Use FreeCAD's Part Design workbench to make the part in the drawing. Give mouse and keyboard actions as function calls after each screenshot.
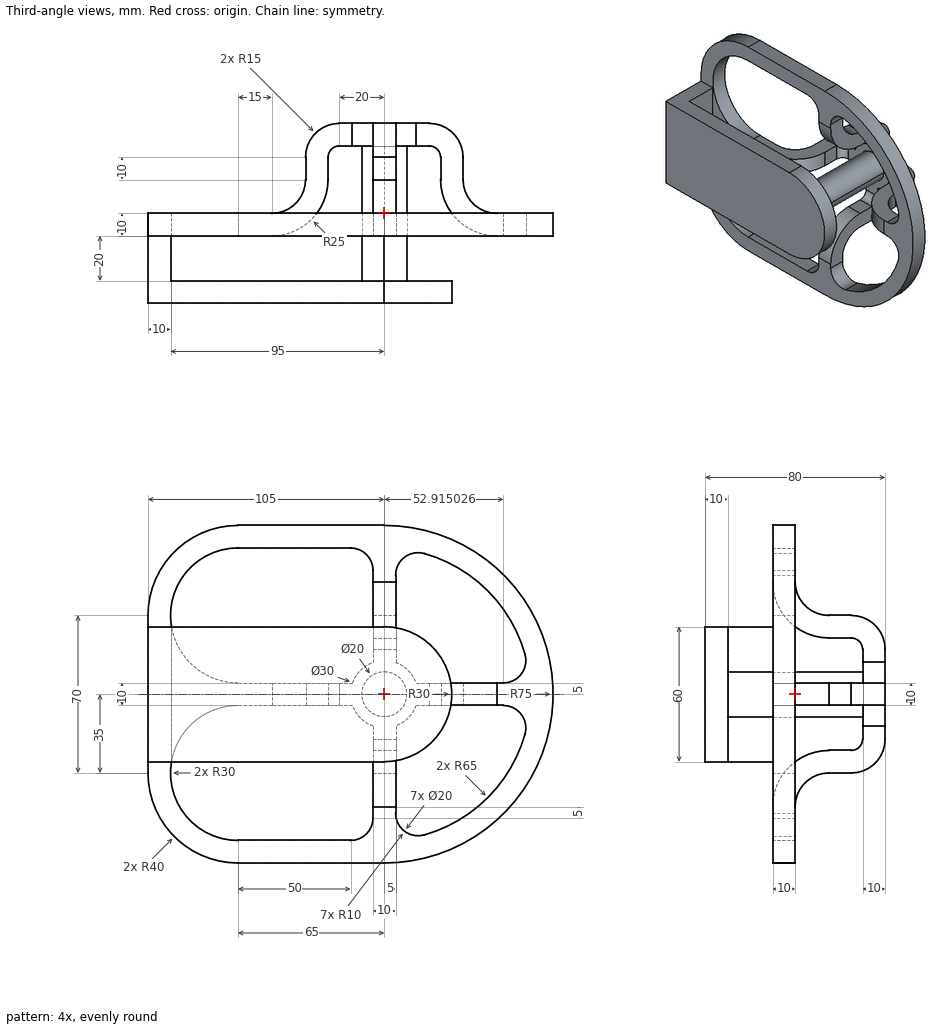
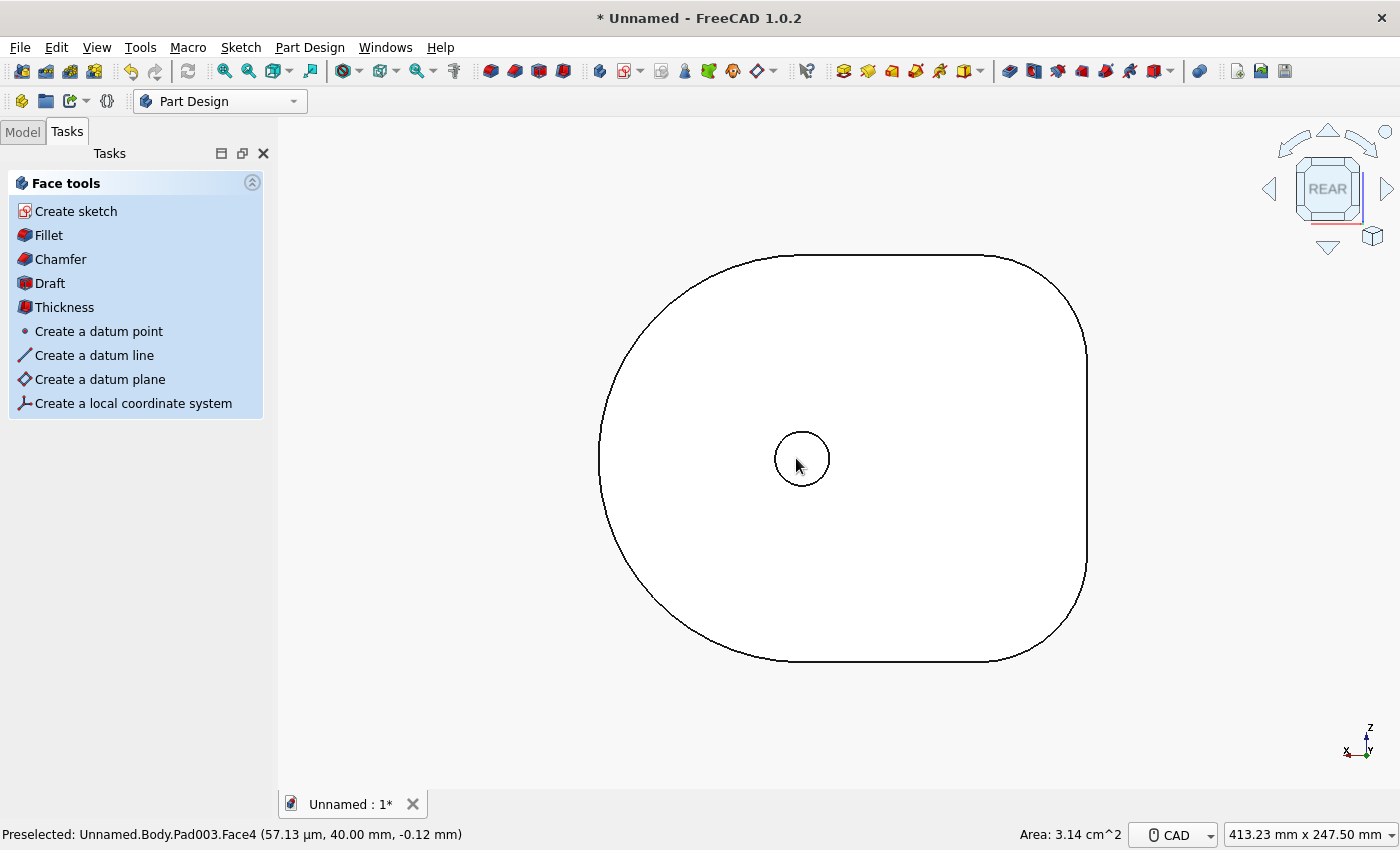
click(624, 72)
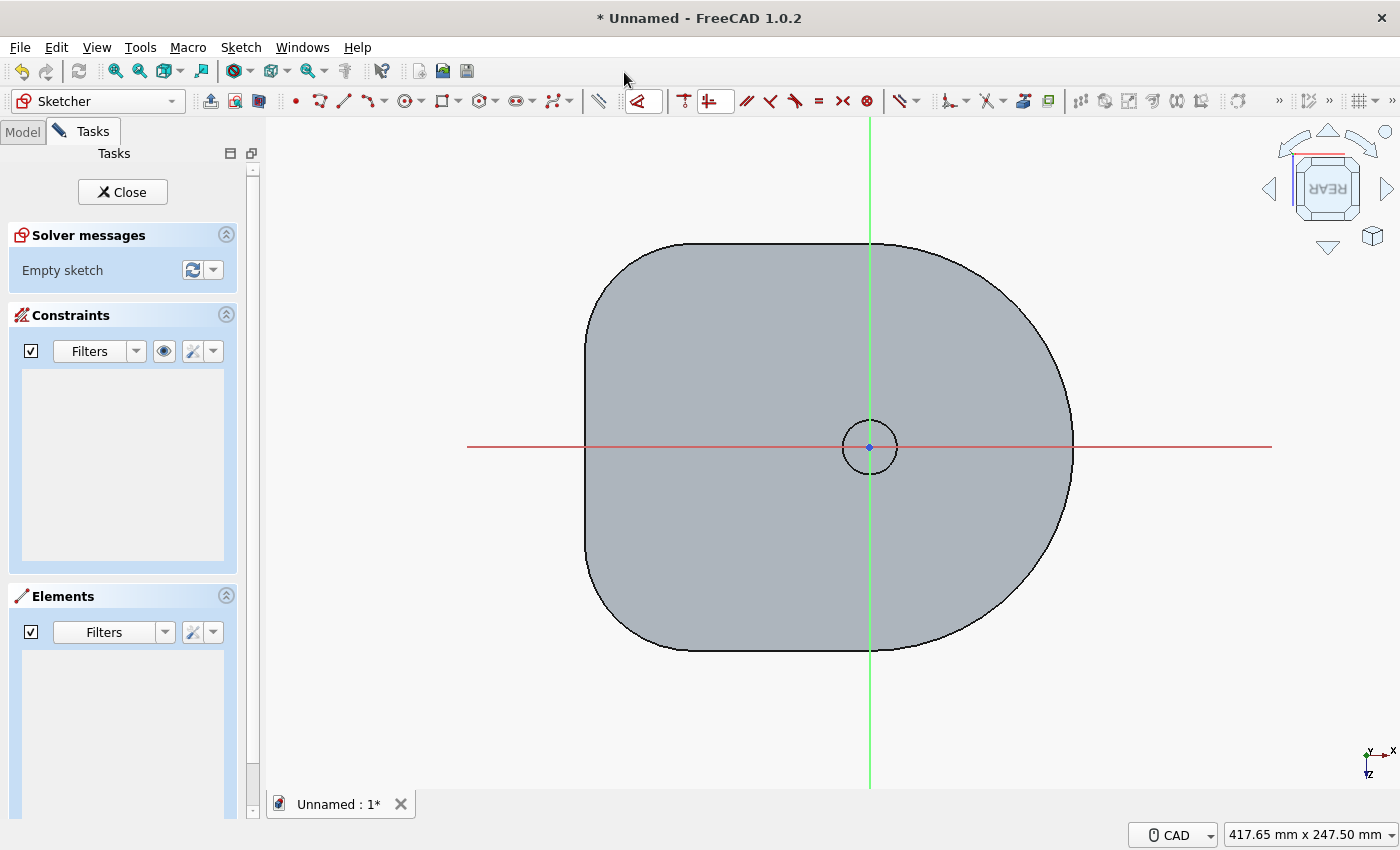
scroll(896, 446, up, 8)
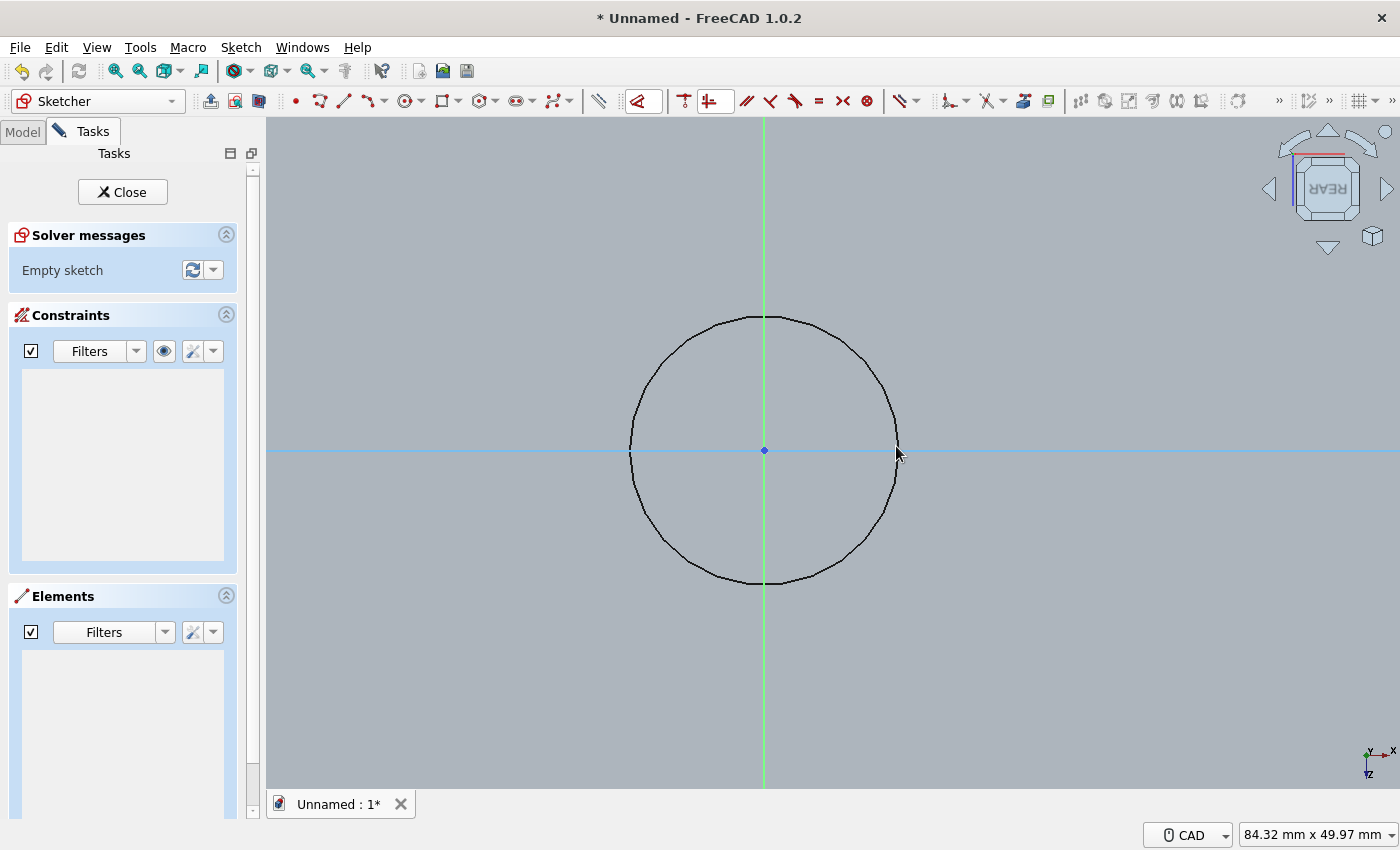
click(406, 102)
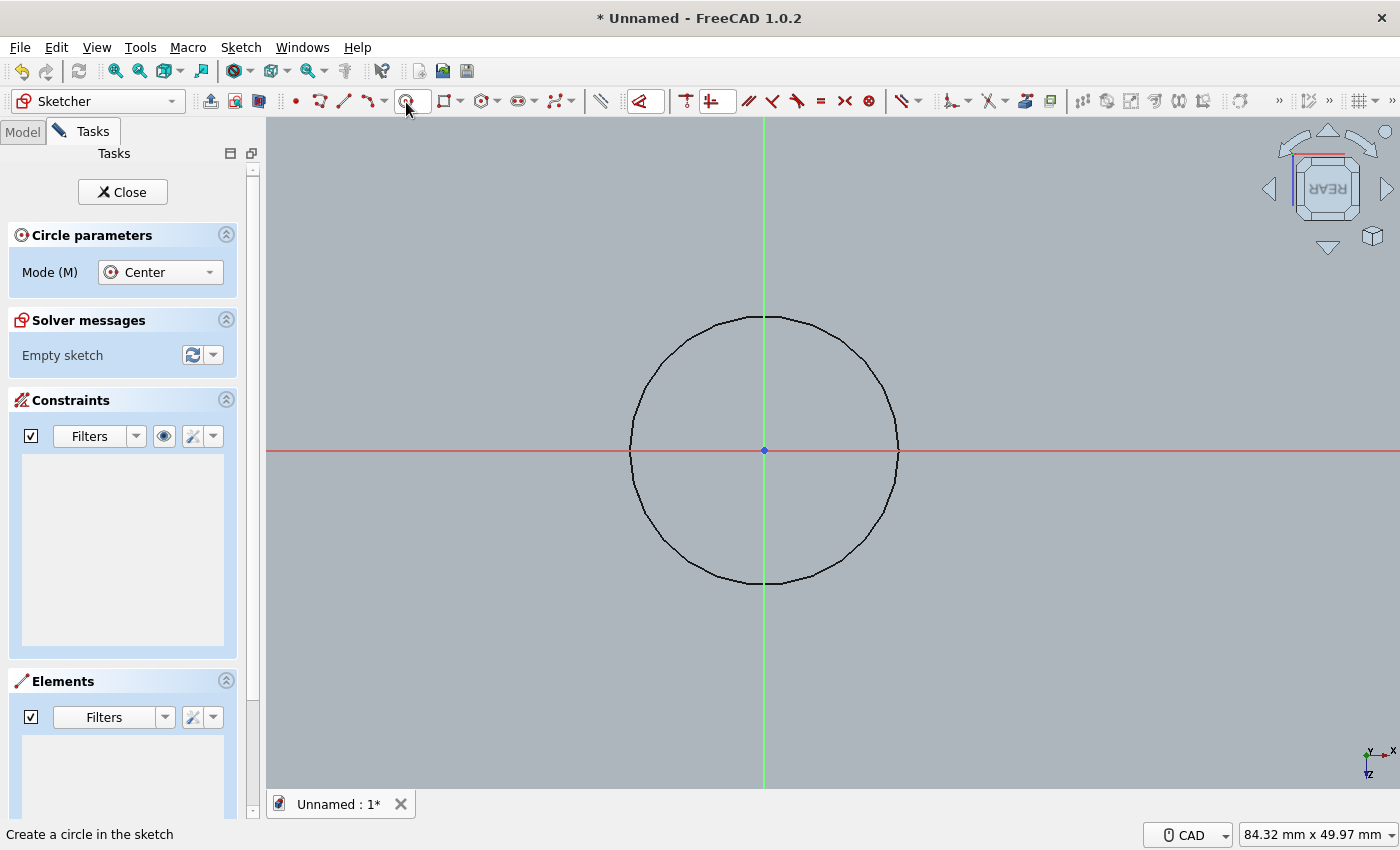
click(764, 451)
move(907, 308)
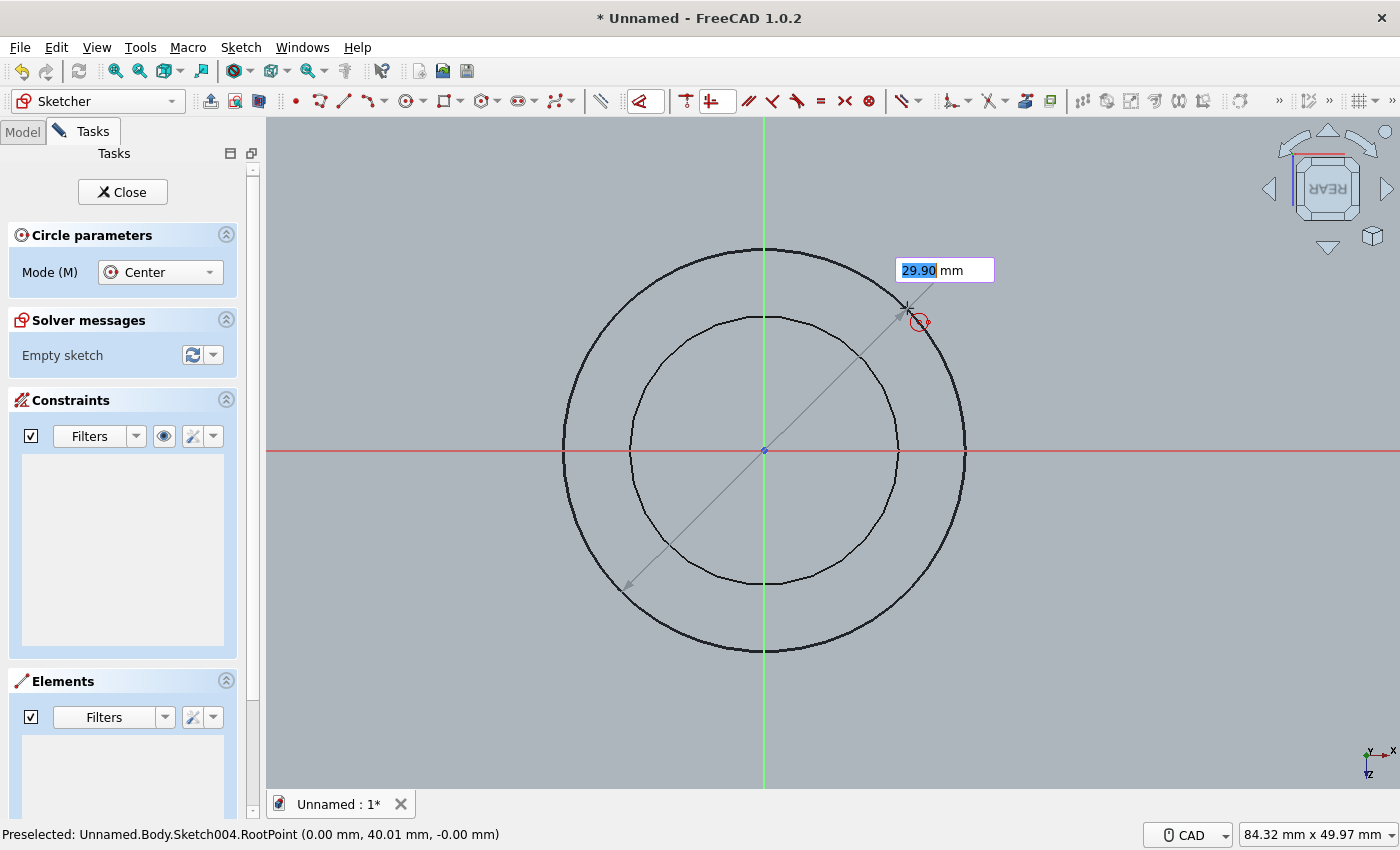
text(30)
key(Return)
key(Escape)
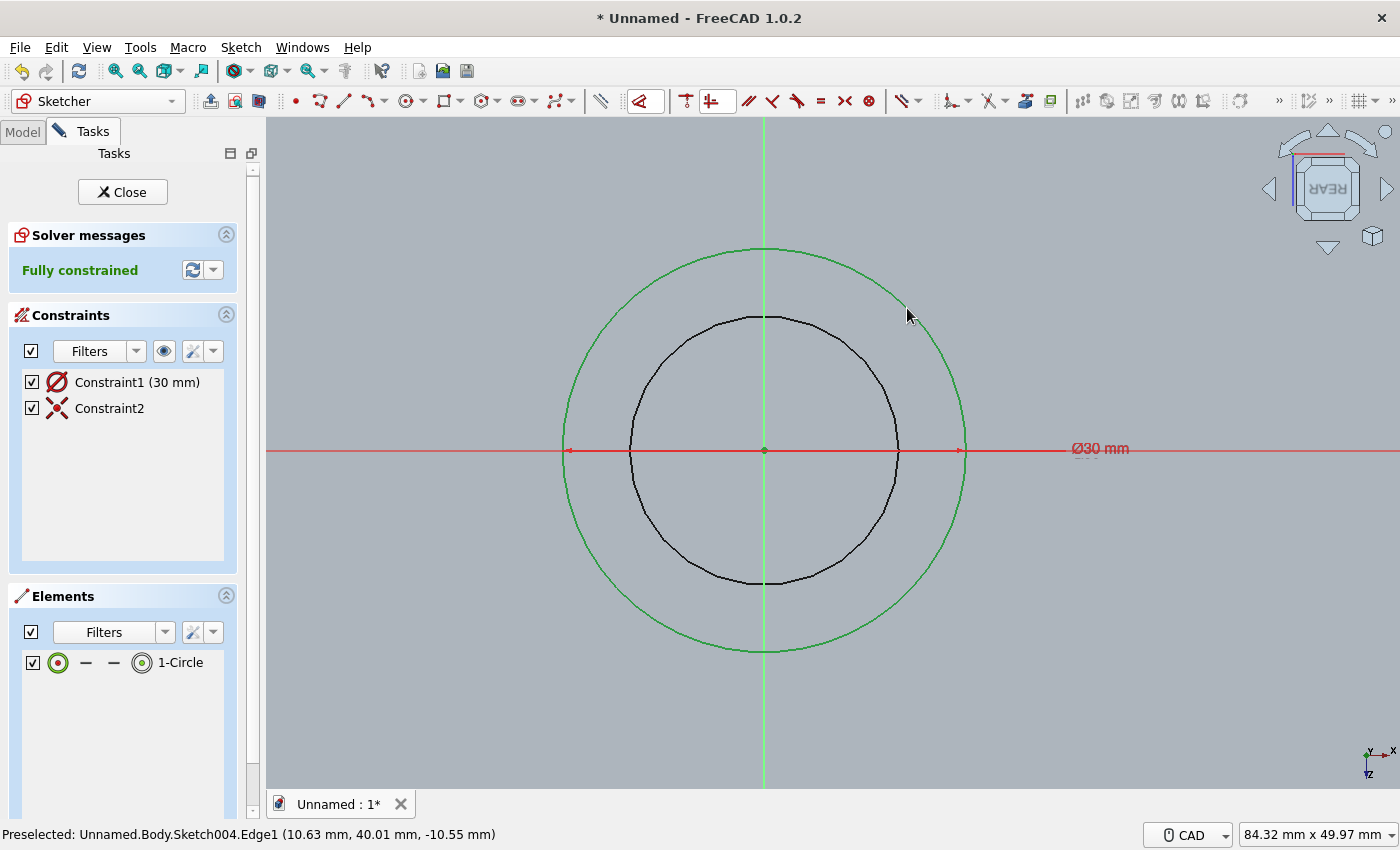
click(123, 192)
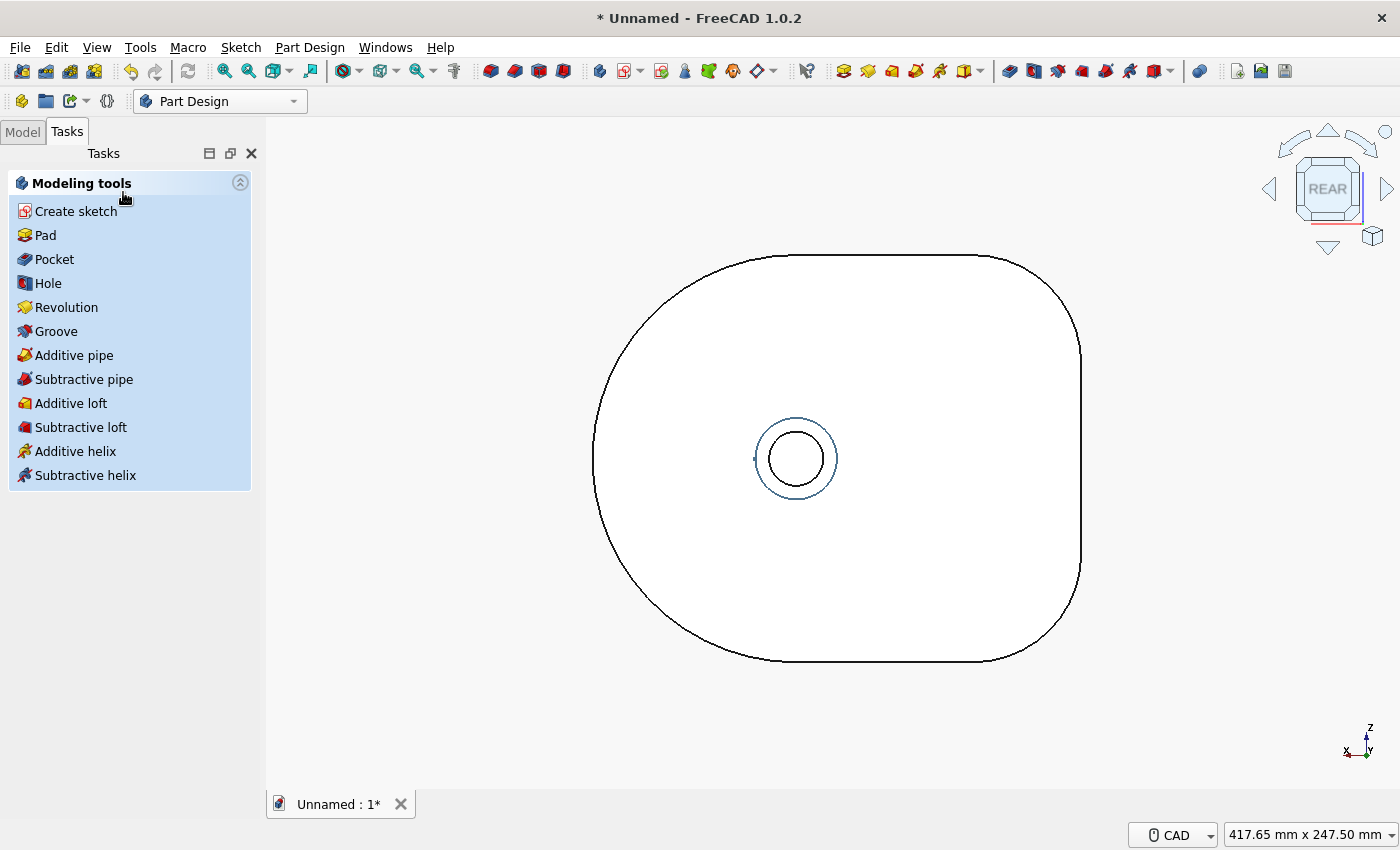
click(844, 72)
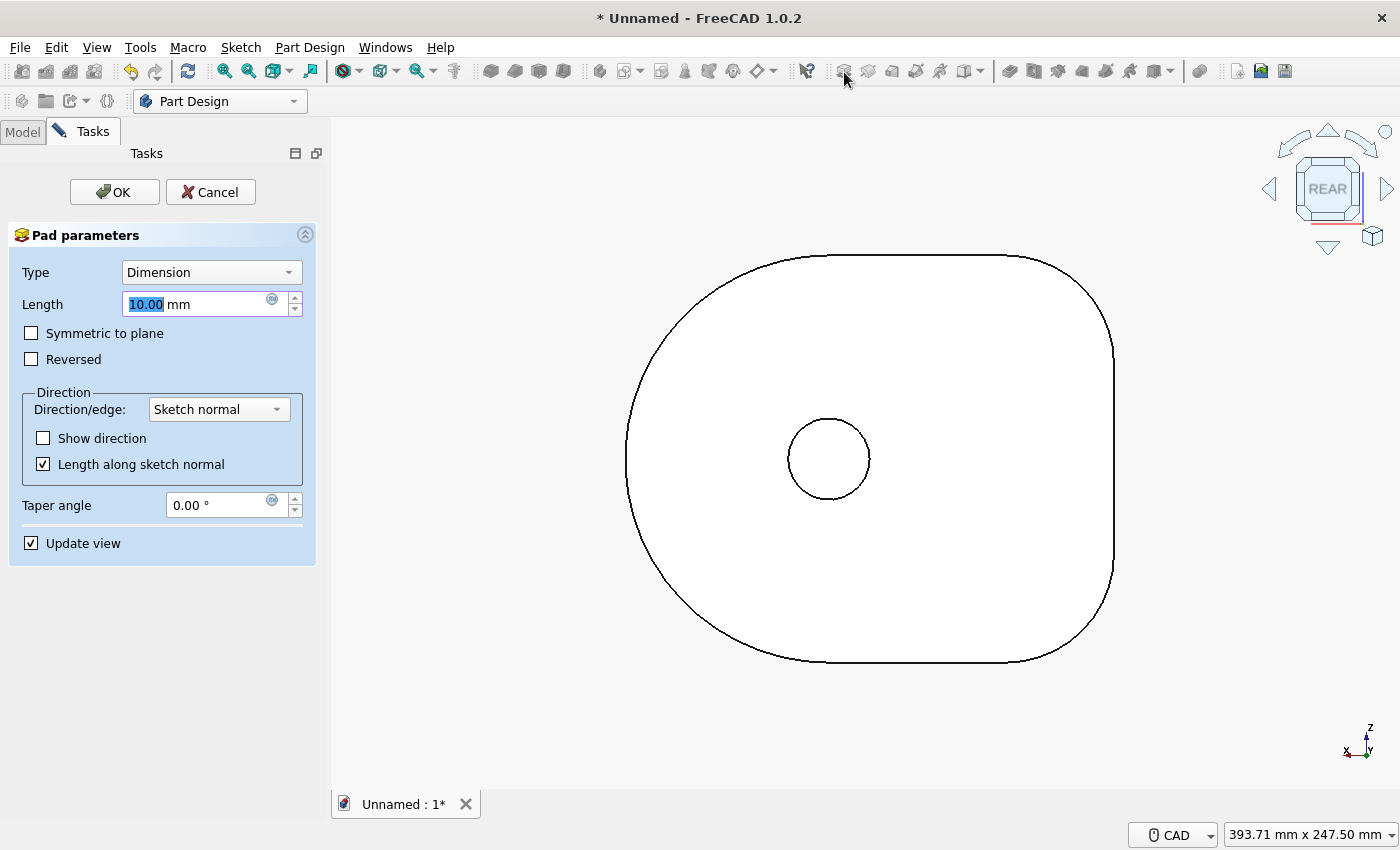
text(10)
key(Tab)